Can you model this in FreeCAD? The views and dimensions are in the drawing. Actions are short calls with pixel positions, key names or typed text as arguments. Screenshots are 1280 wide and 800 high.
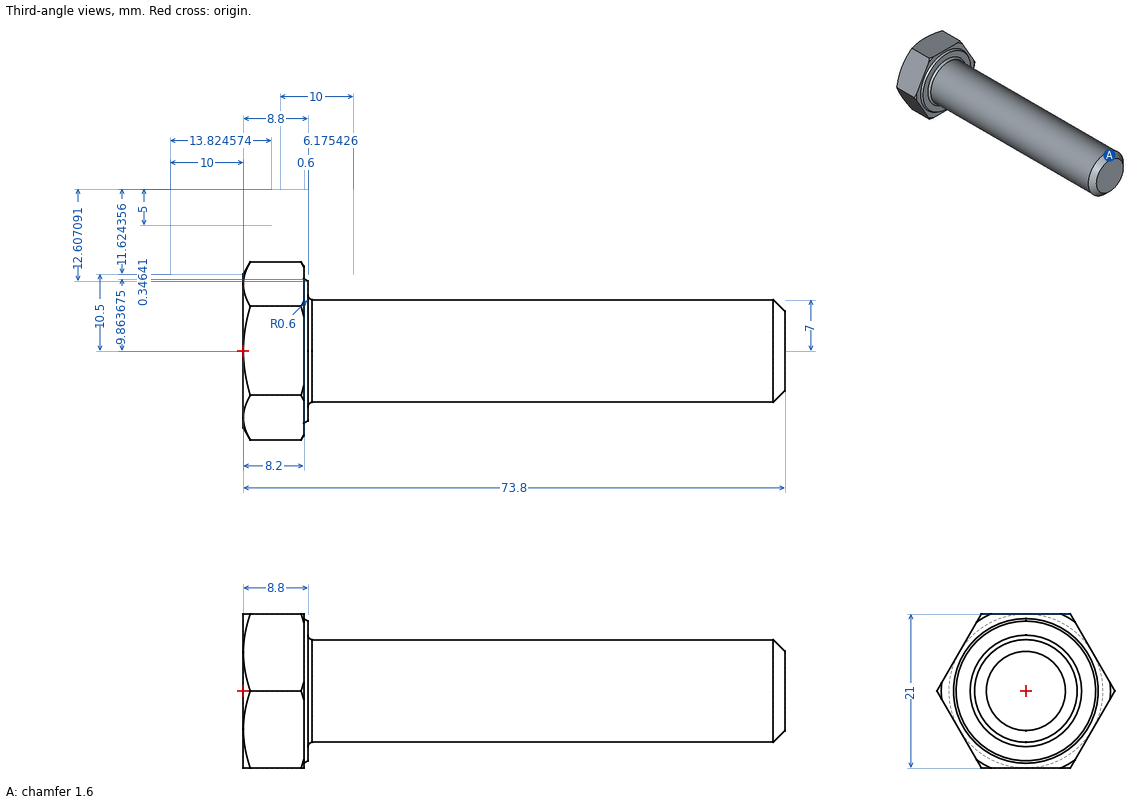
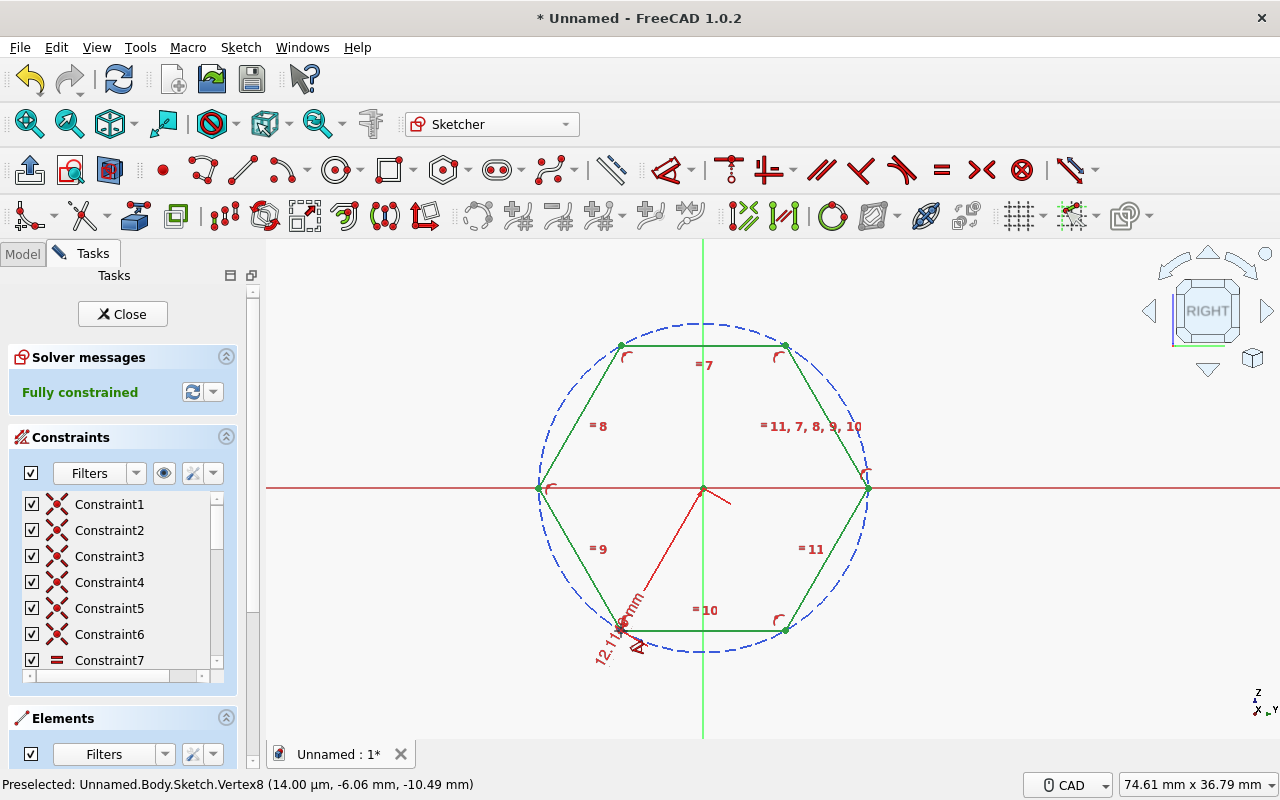
click(786, 346)
click(539, 388)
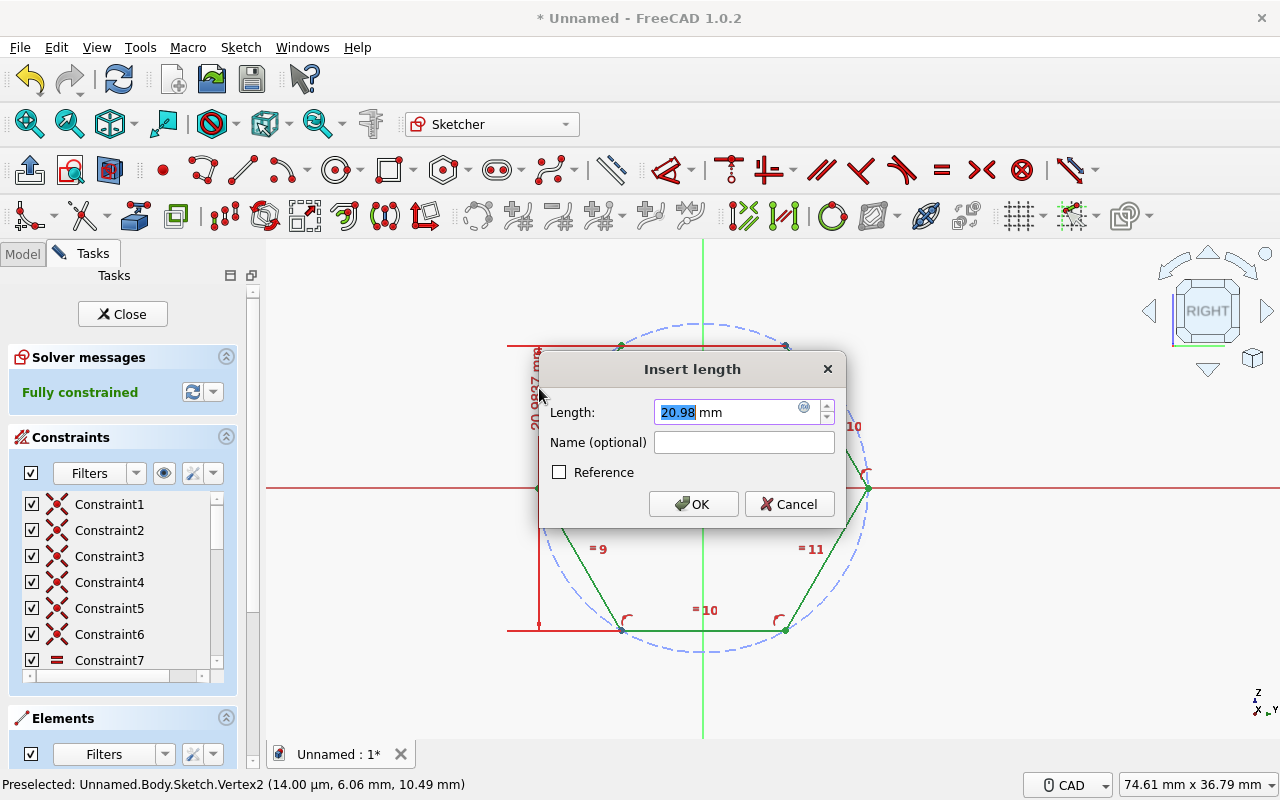
text(21)
key(Return)
key(Escape)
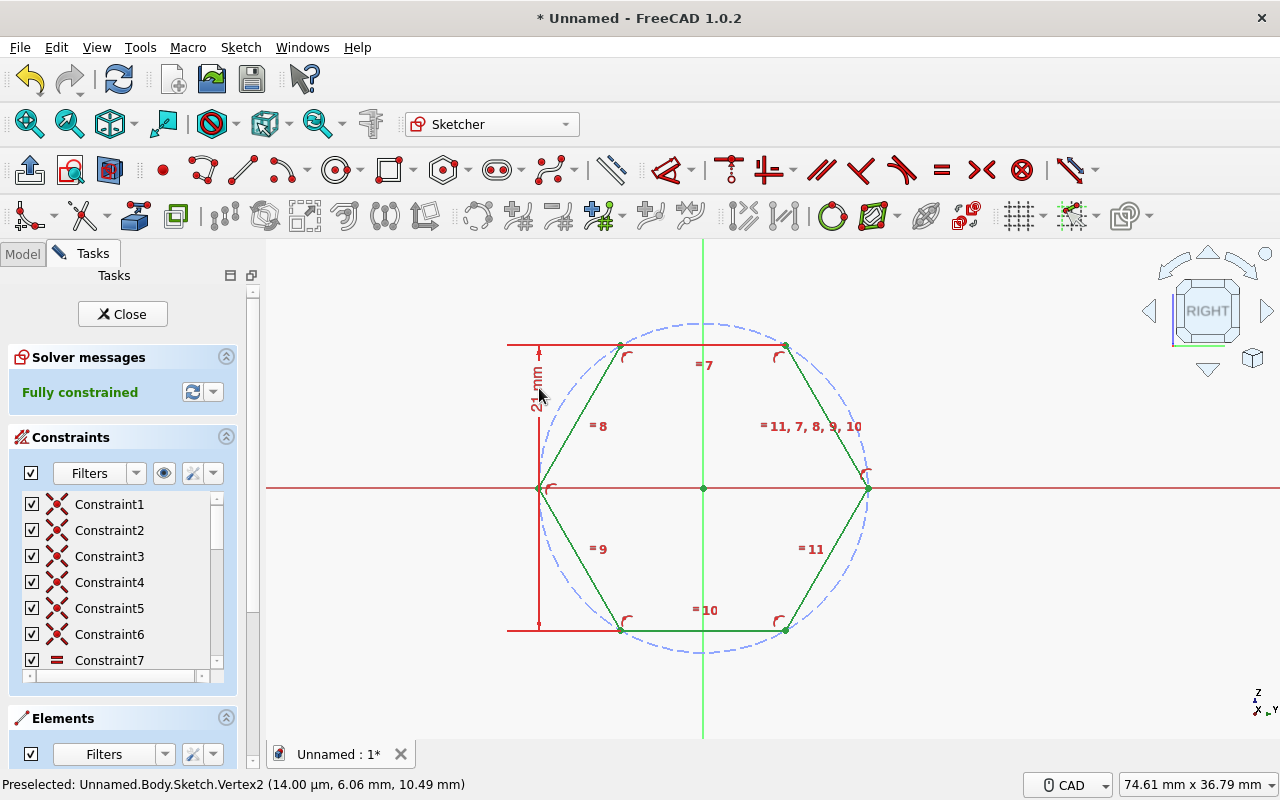
click(123, 314)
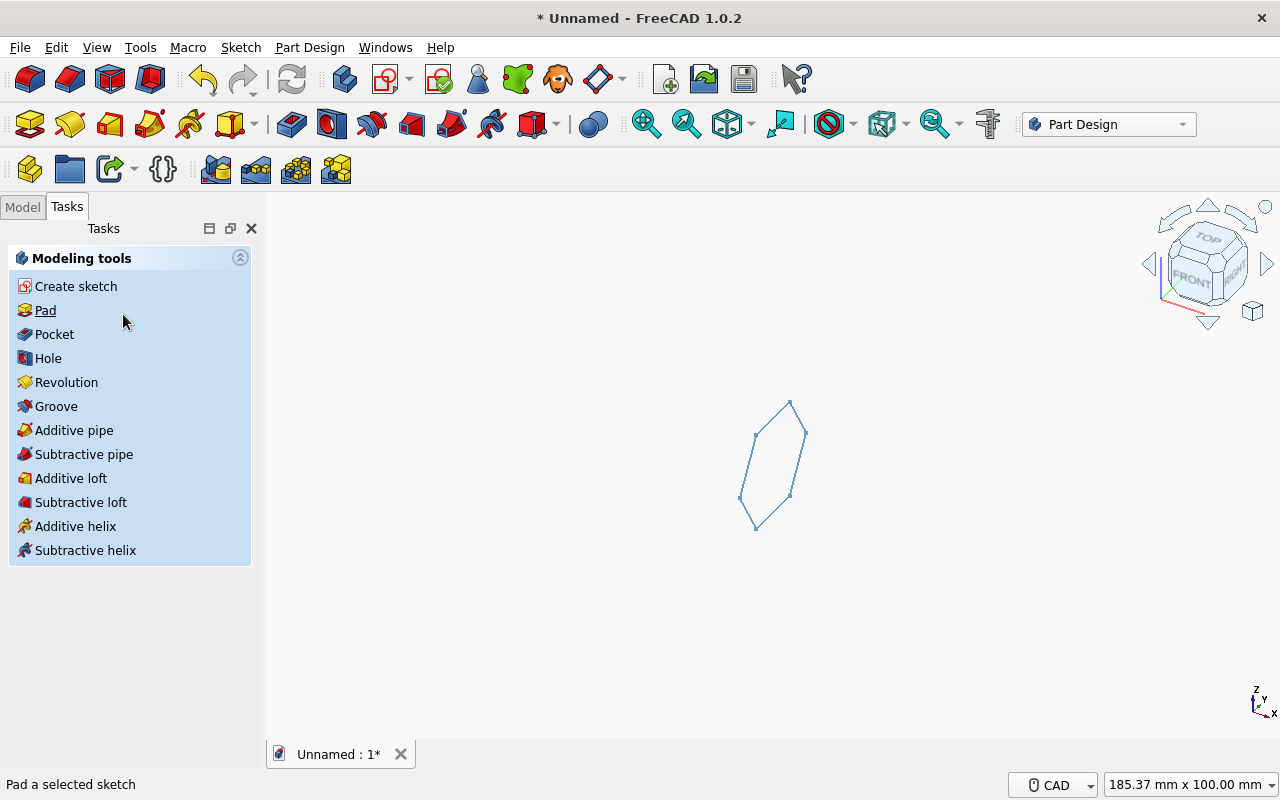
click(30, 124)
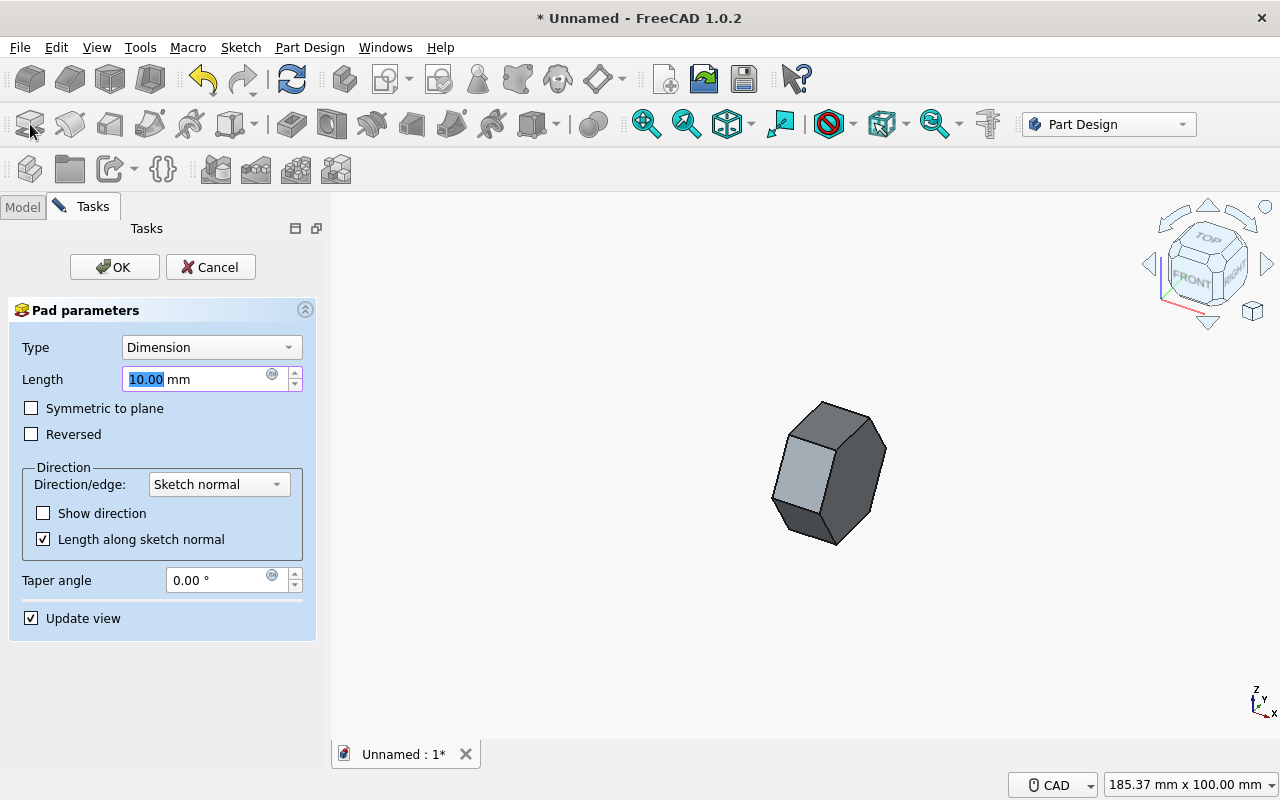
text(8.8)
key(Tab)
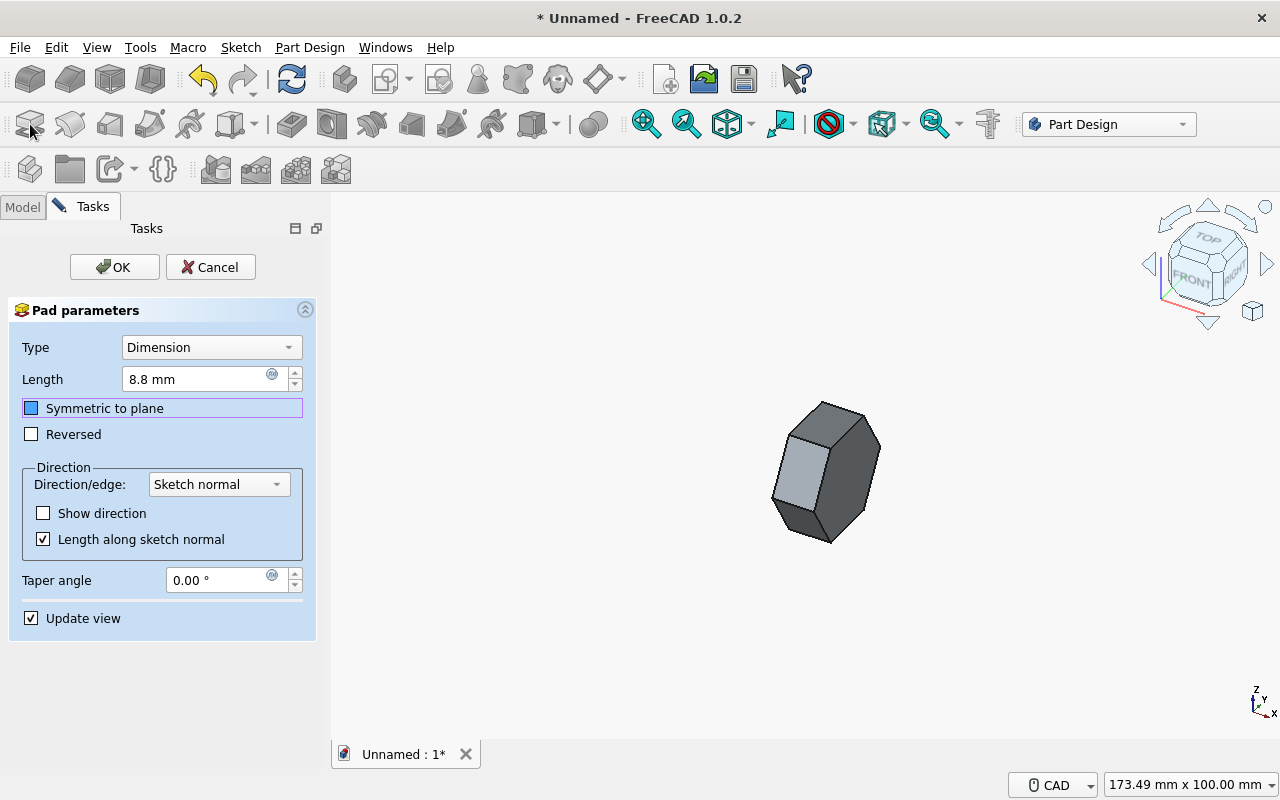
click(115, 267)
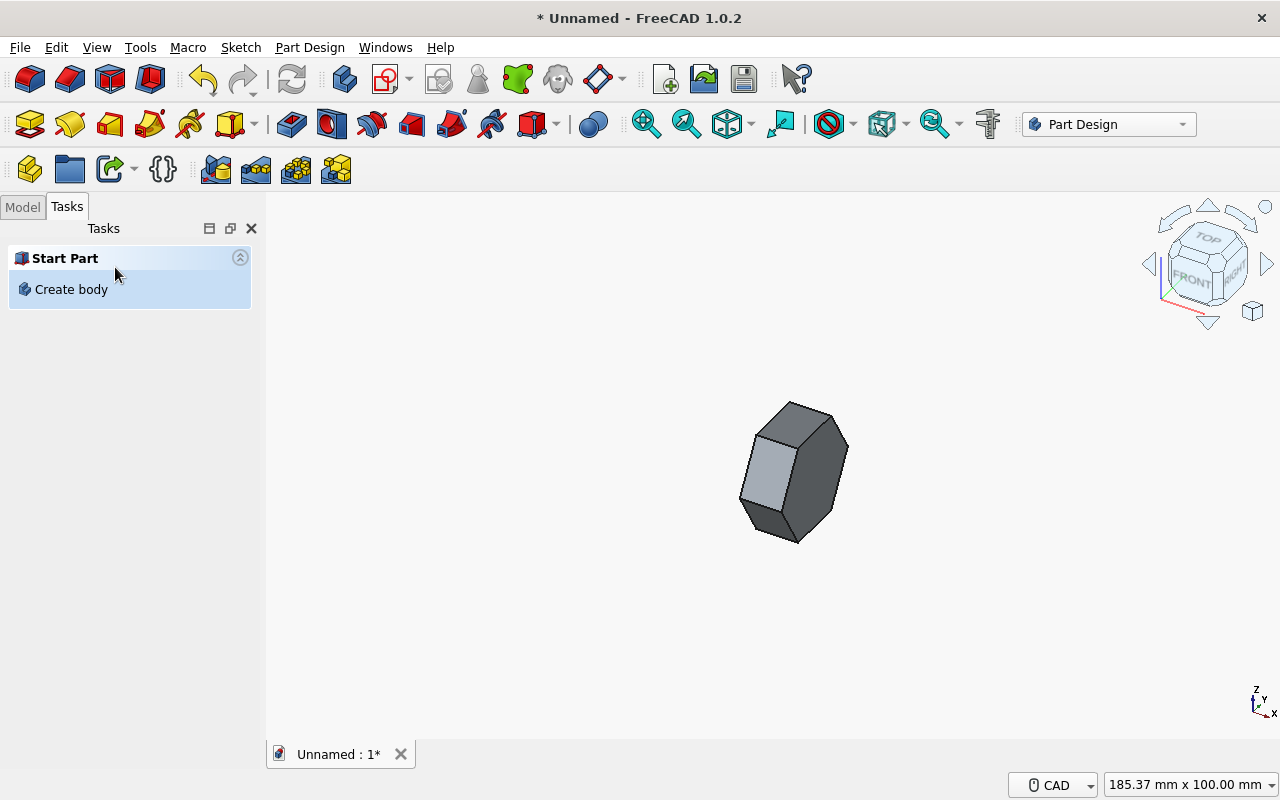
click(648, 124)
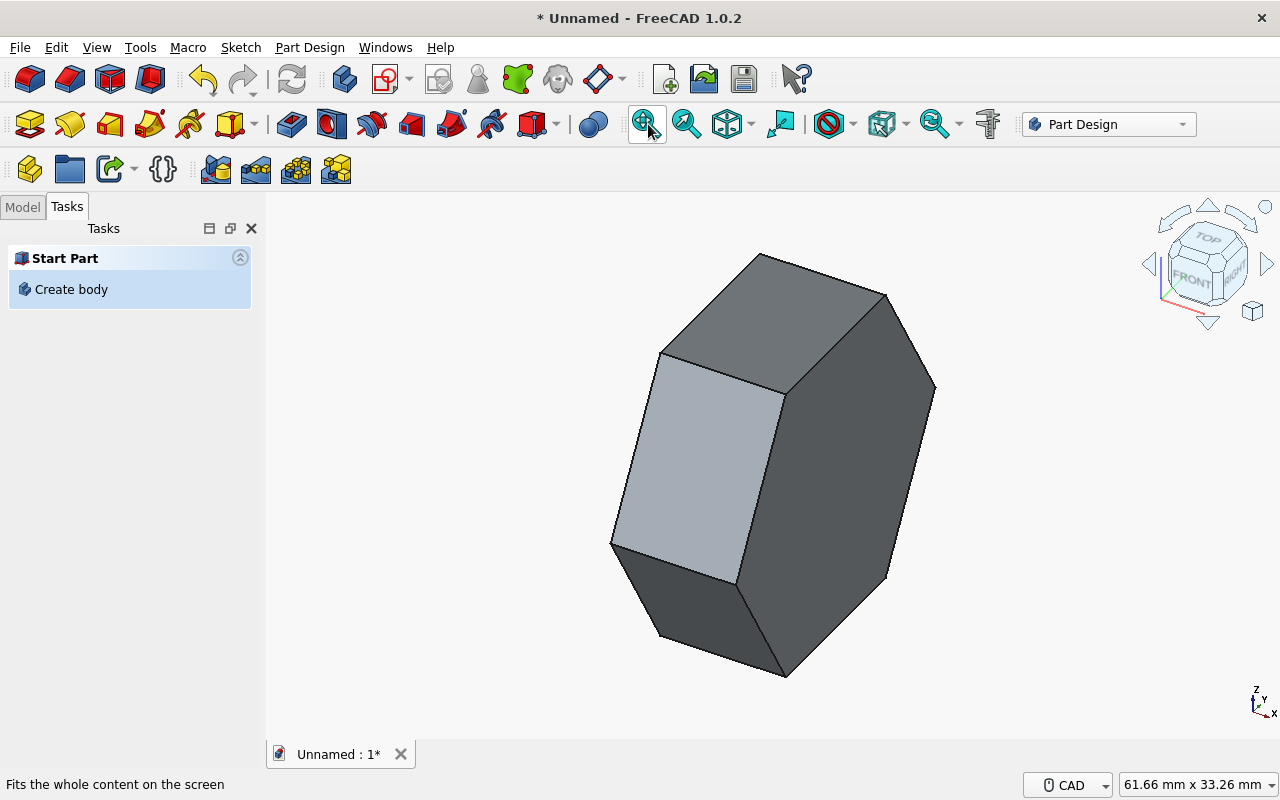
click(386, 80)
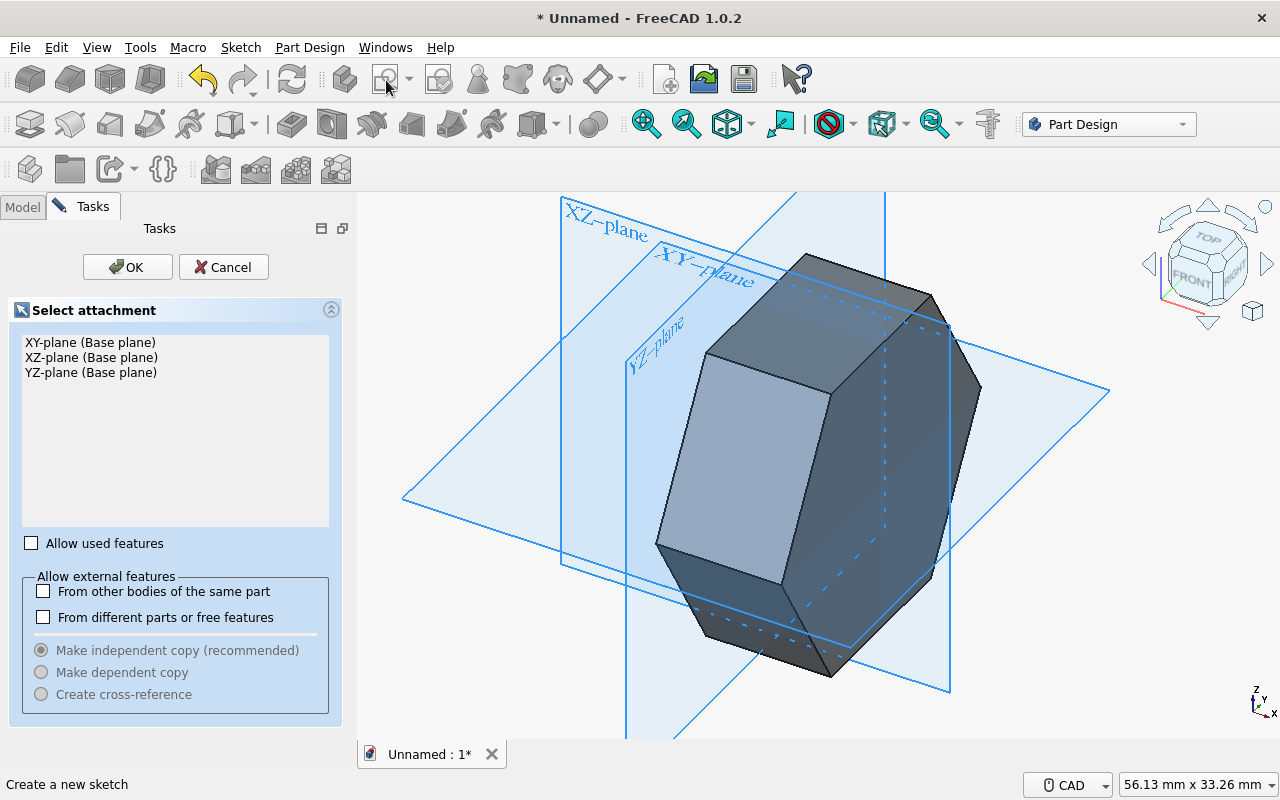
click(82, 342)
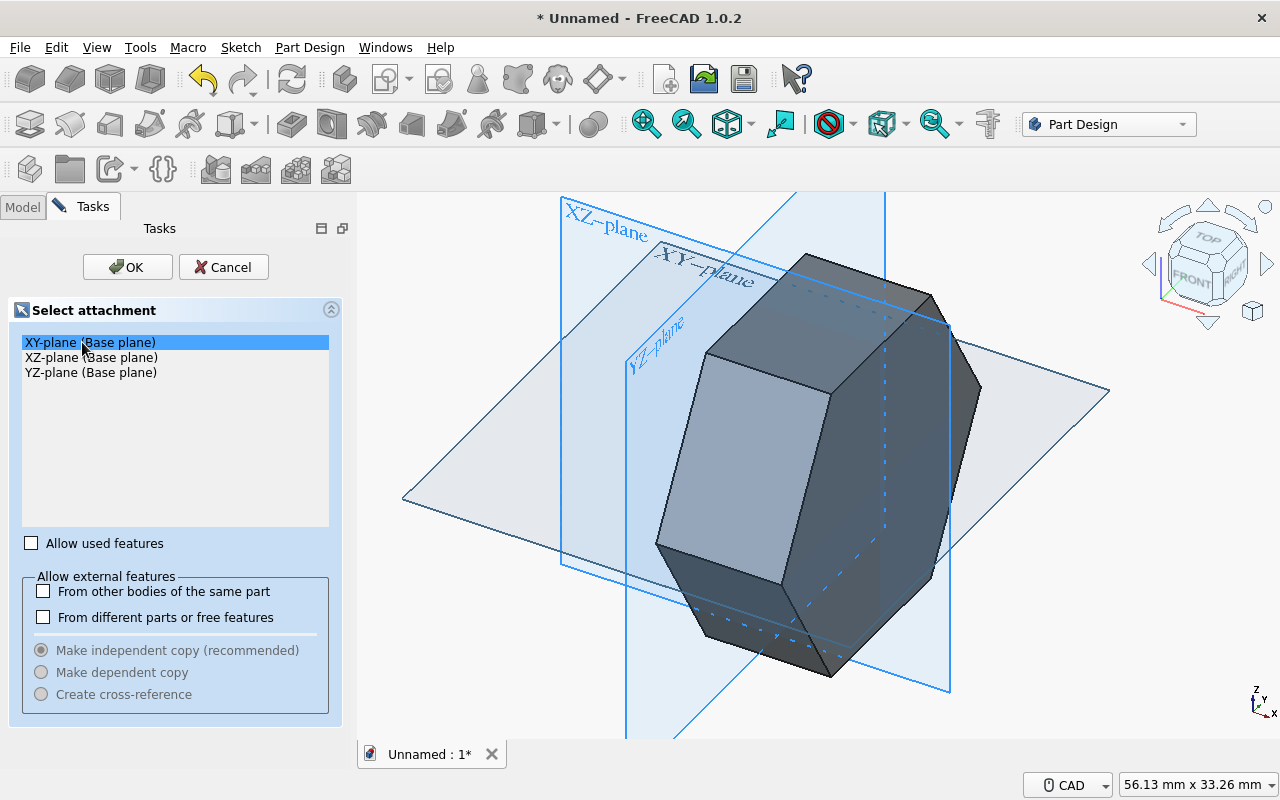
click(128, 267)